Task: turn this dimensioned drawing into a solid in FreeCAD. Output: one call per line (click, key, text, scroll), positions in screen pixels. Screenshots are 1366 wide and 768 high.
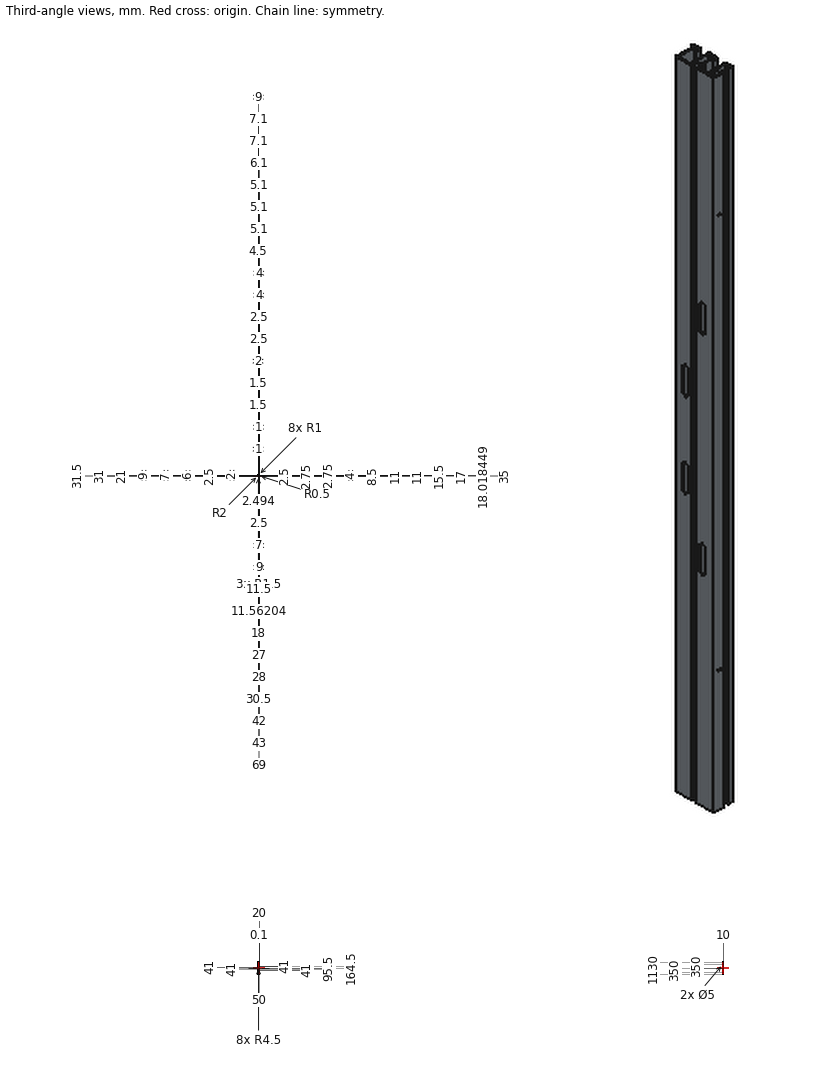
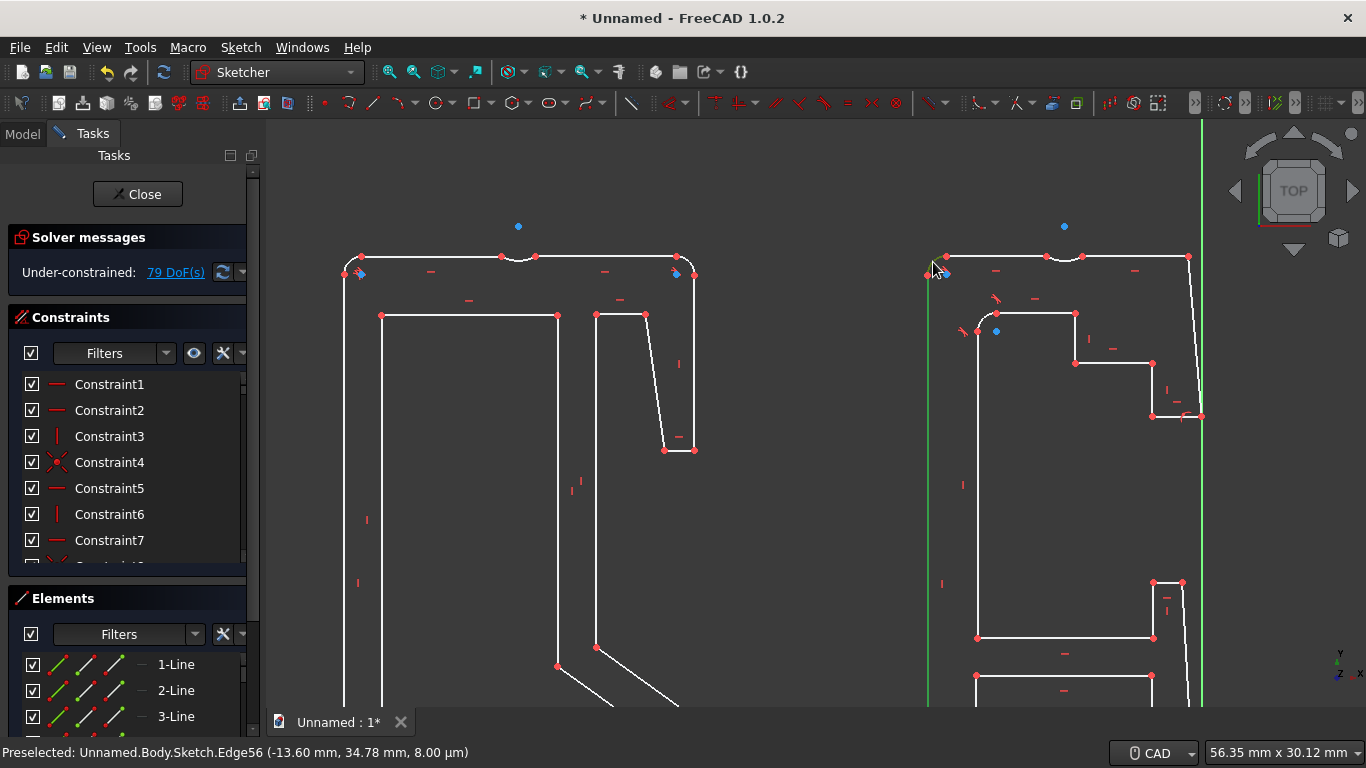
click(824, 104)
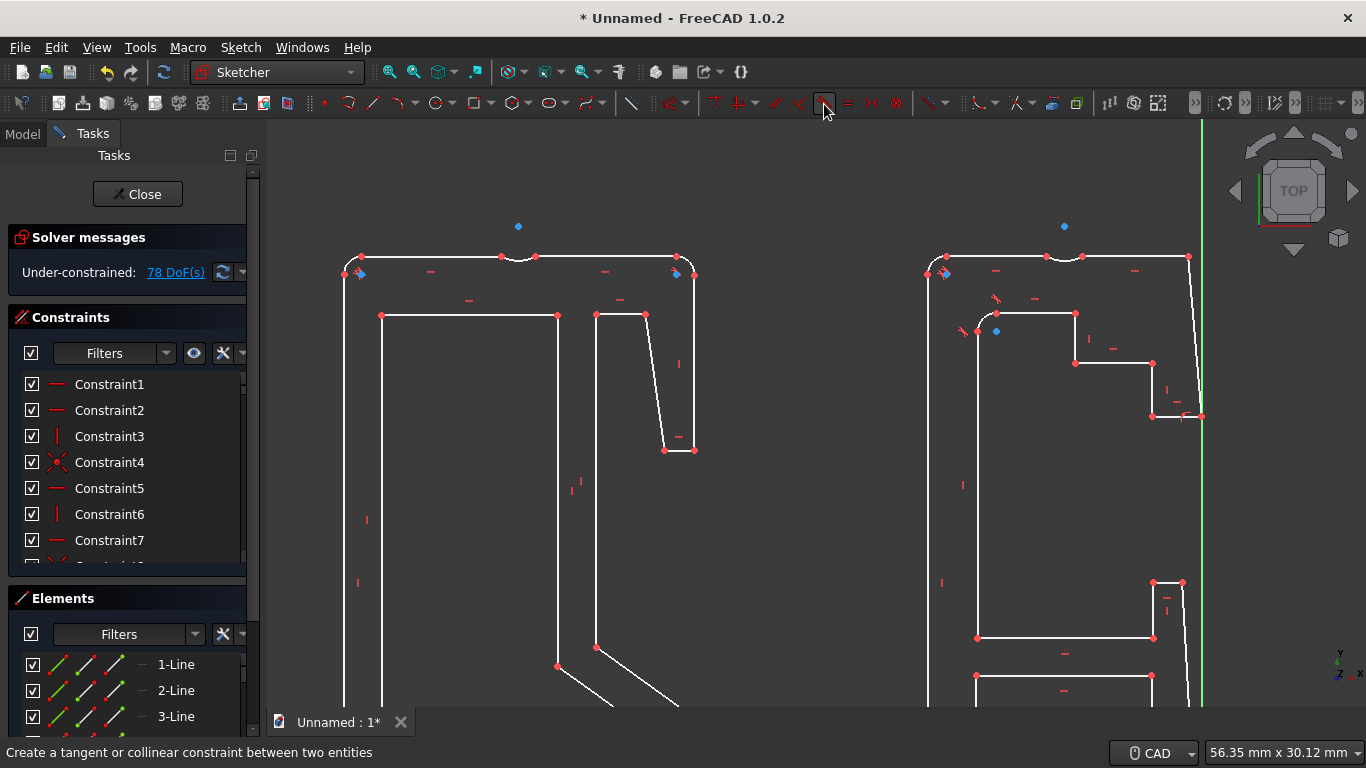
click(694, 398)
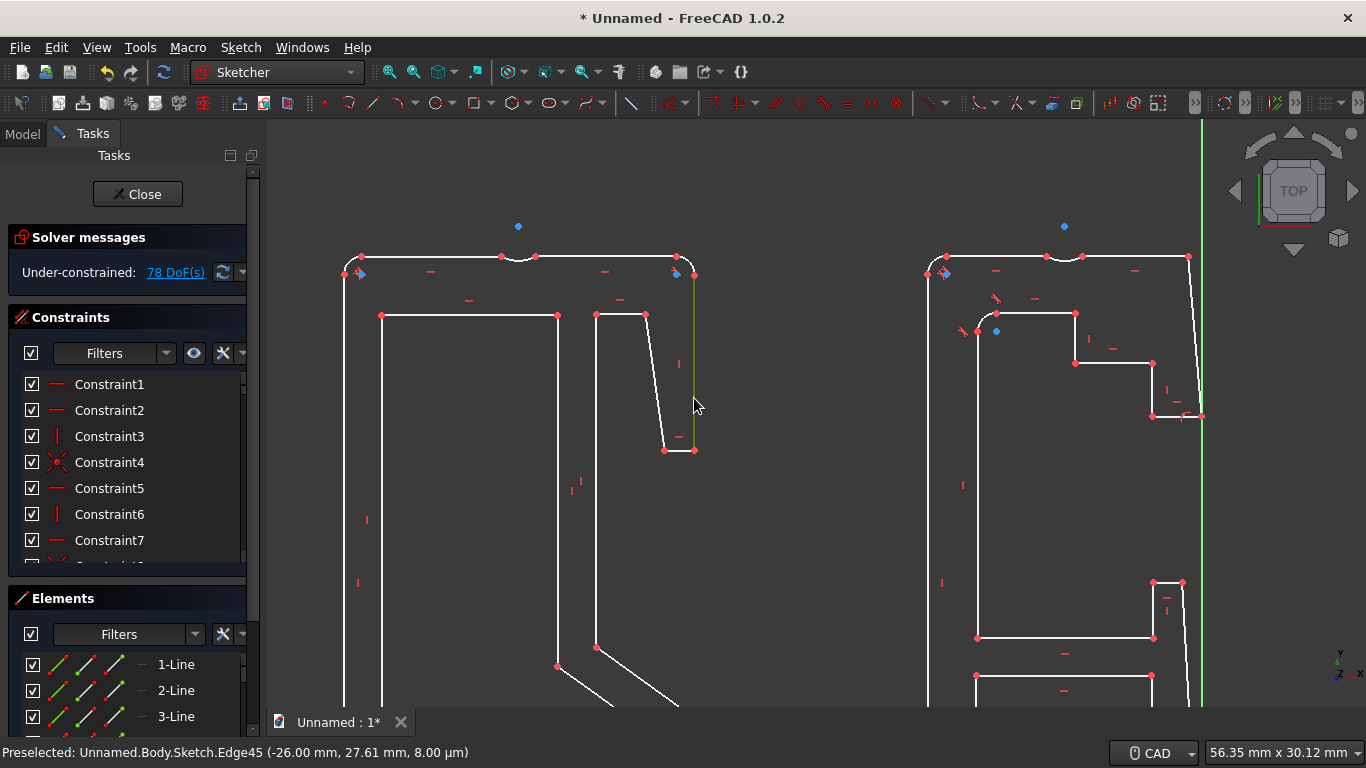
click(690, 262)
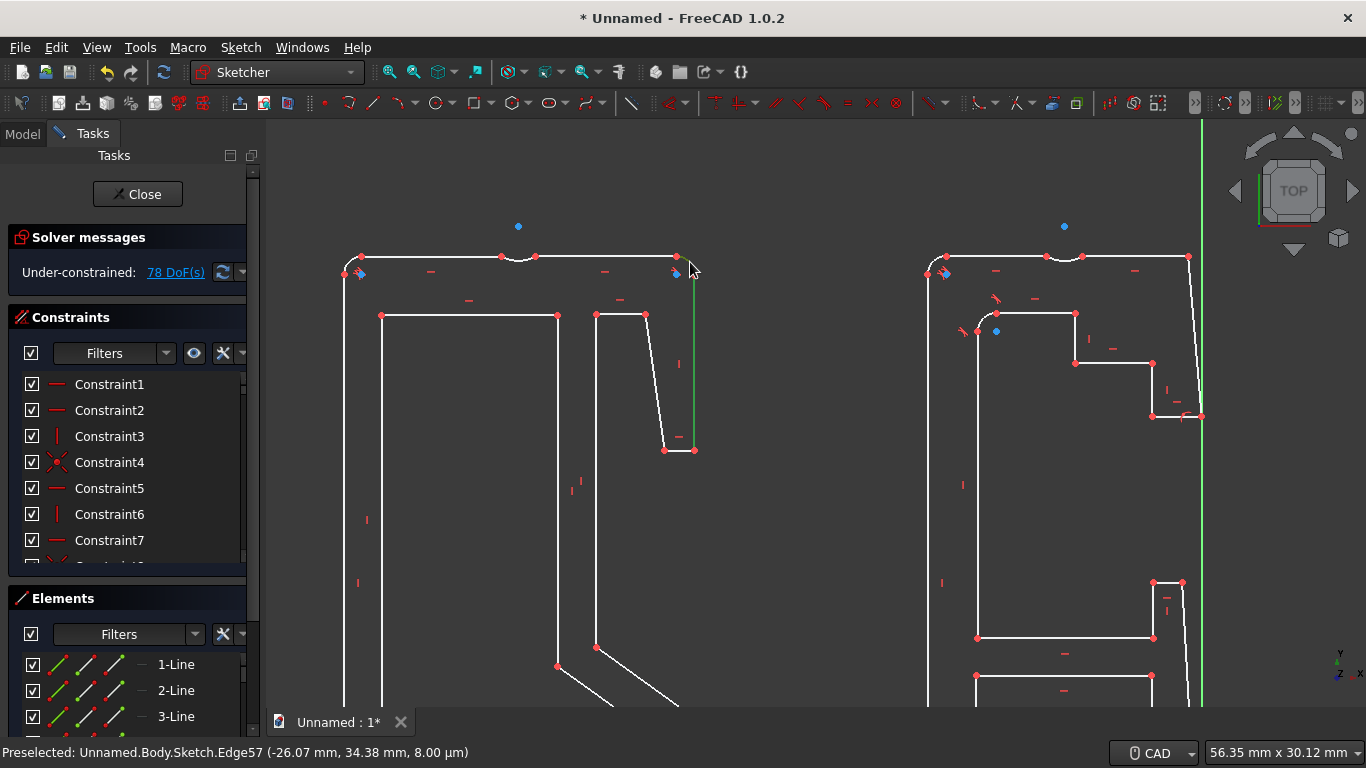
key(t)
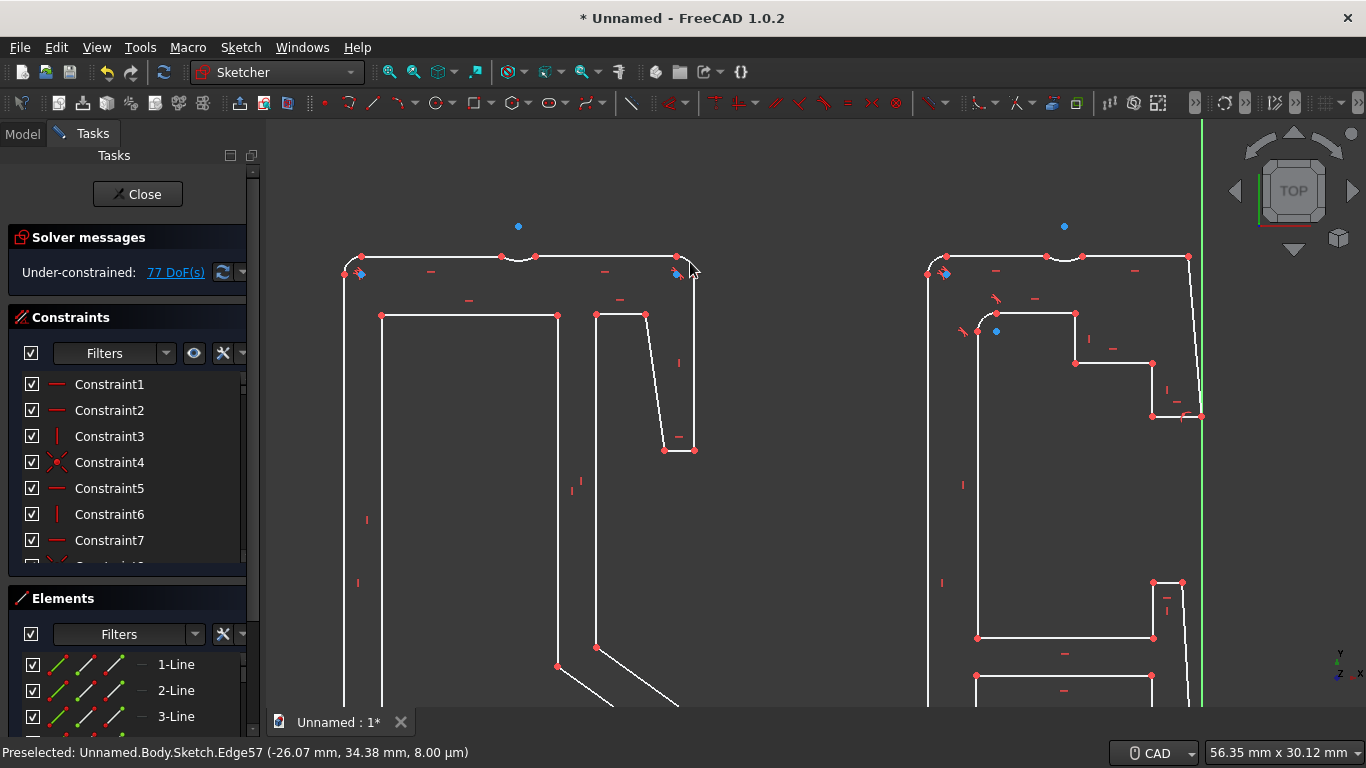
scroll(934, 263, down, 4)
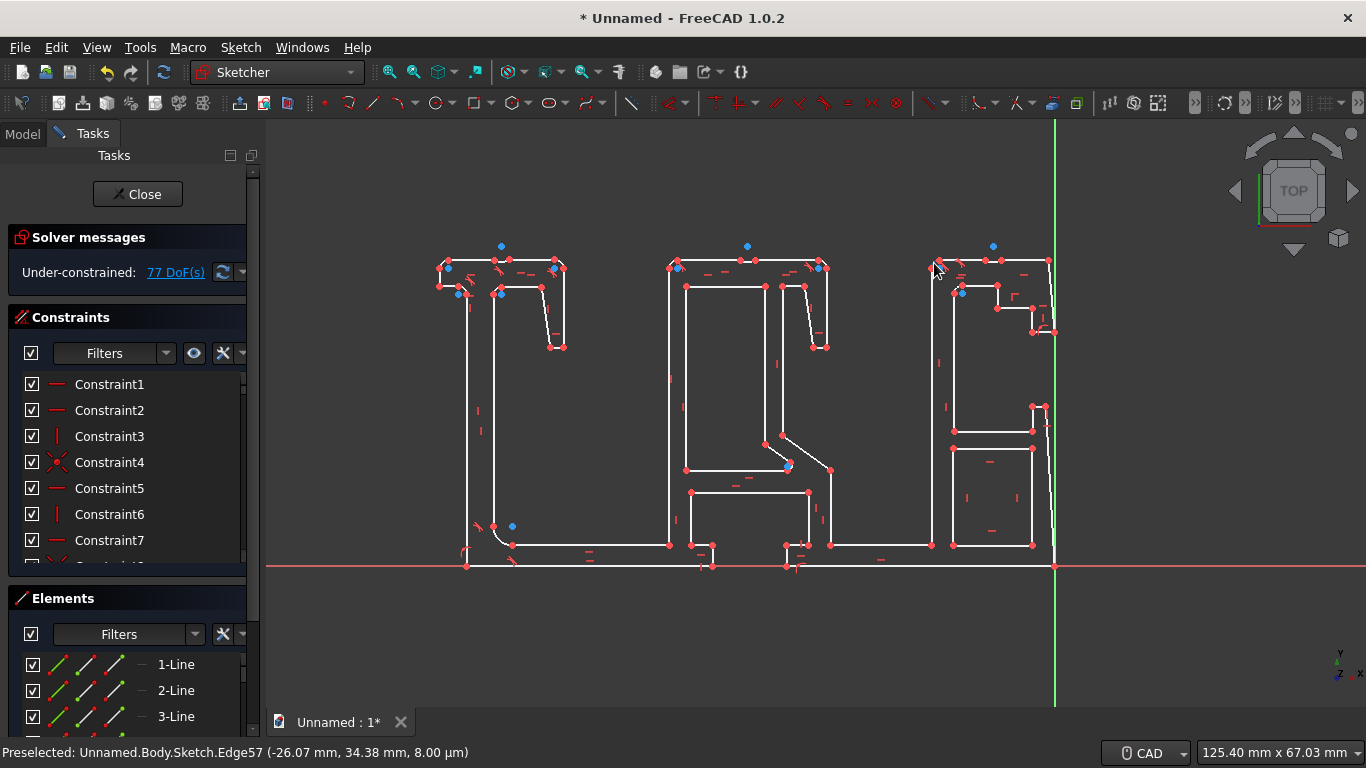
click(757, 471)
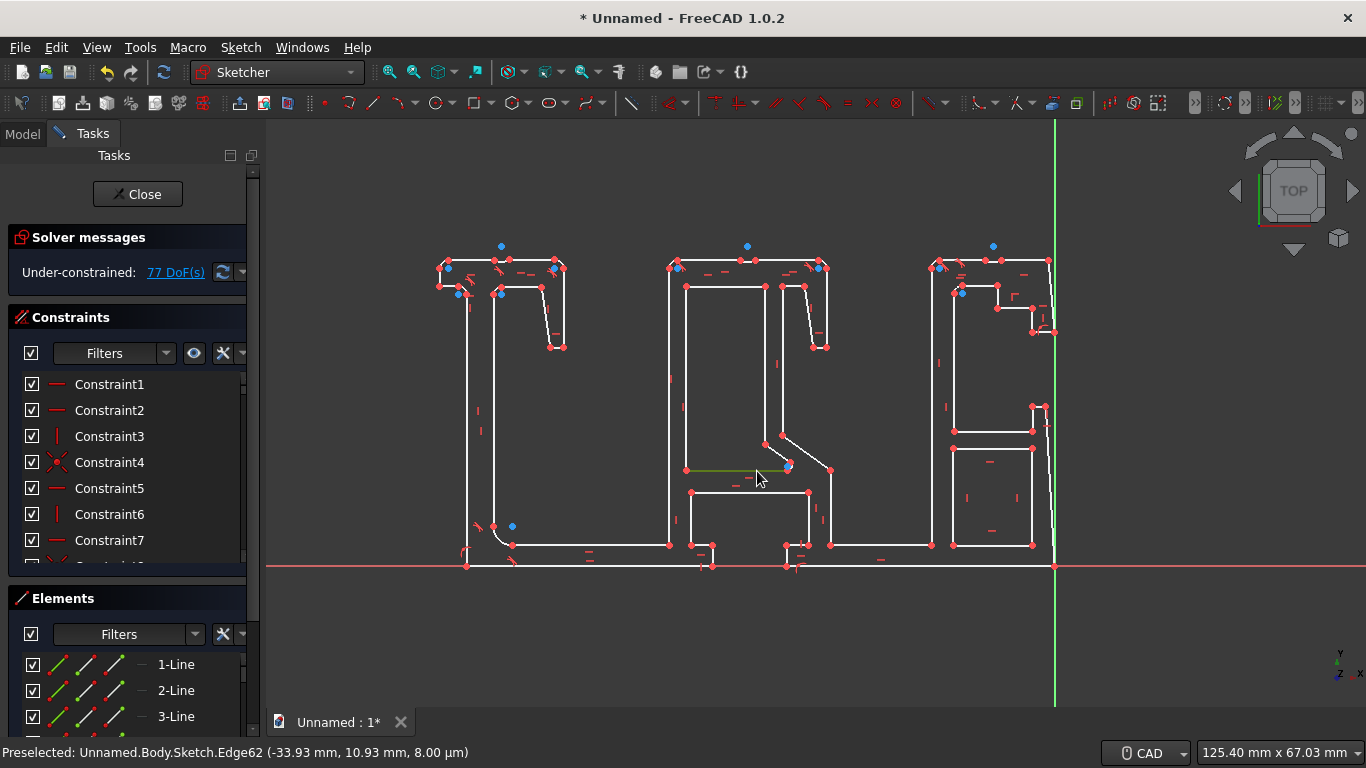
scroll(792, 467, up, 6)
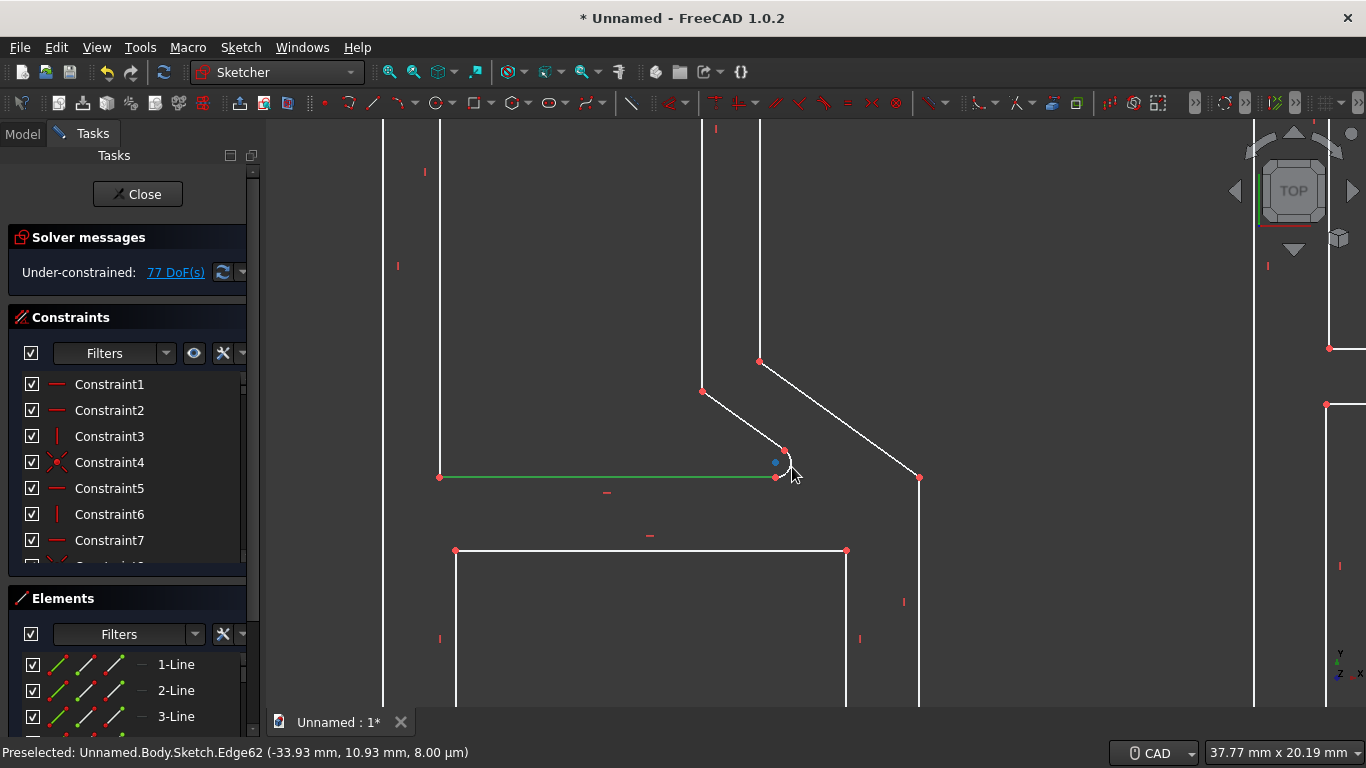
click(790, 467)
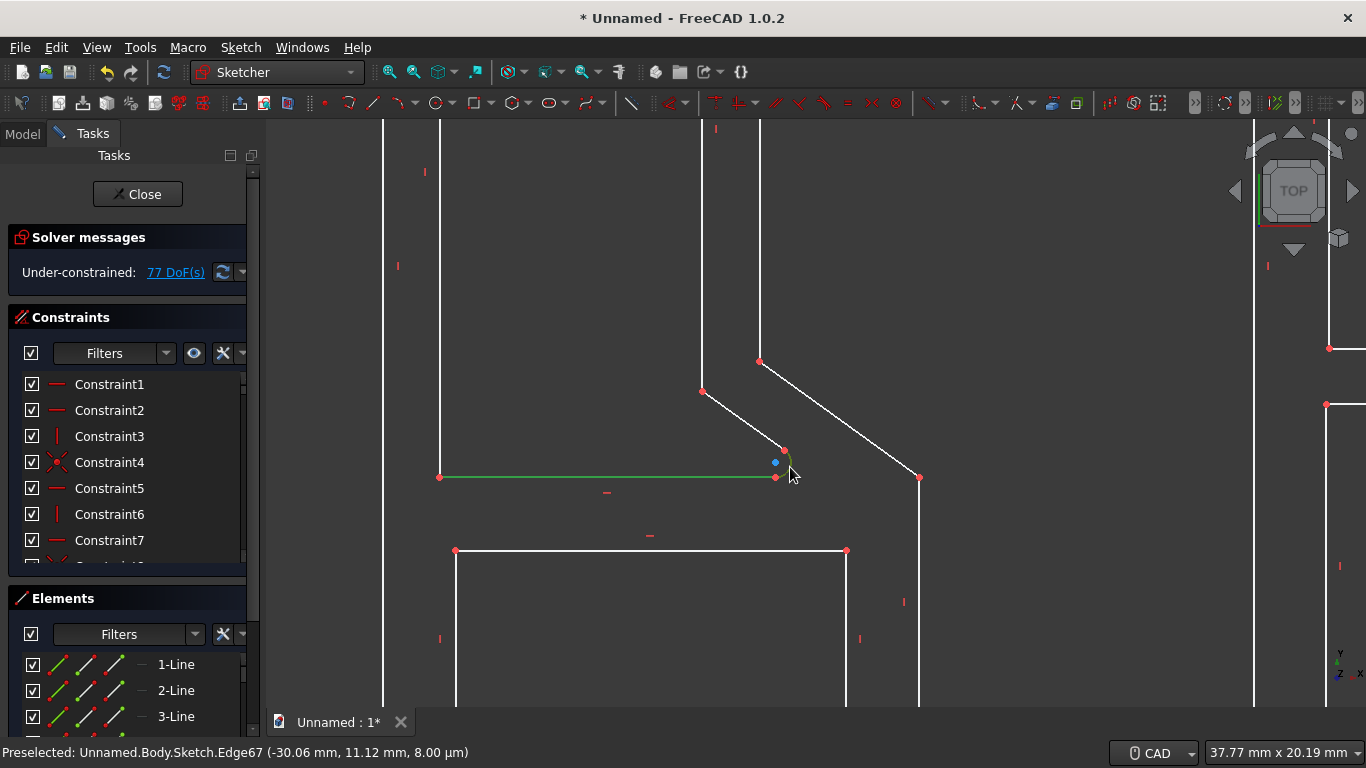
key(t)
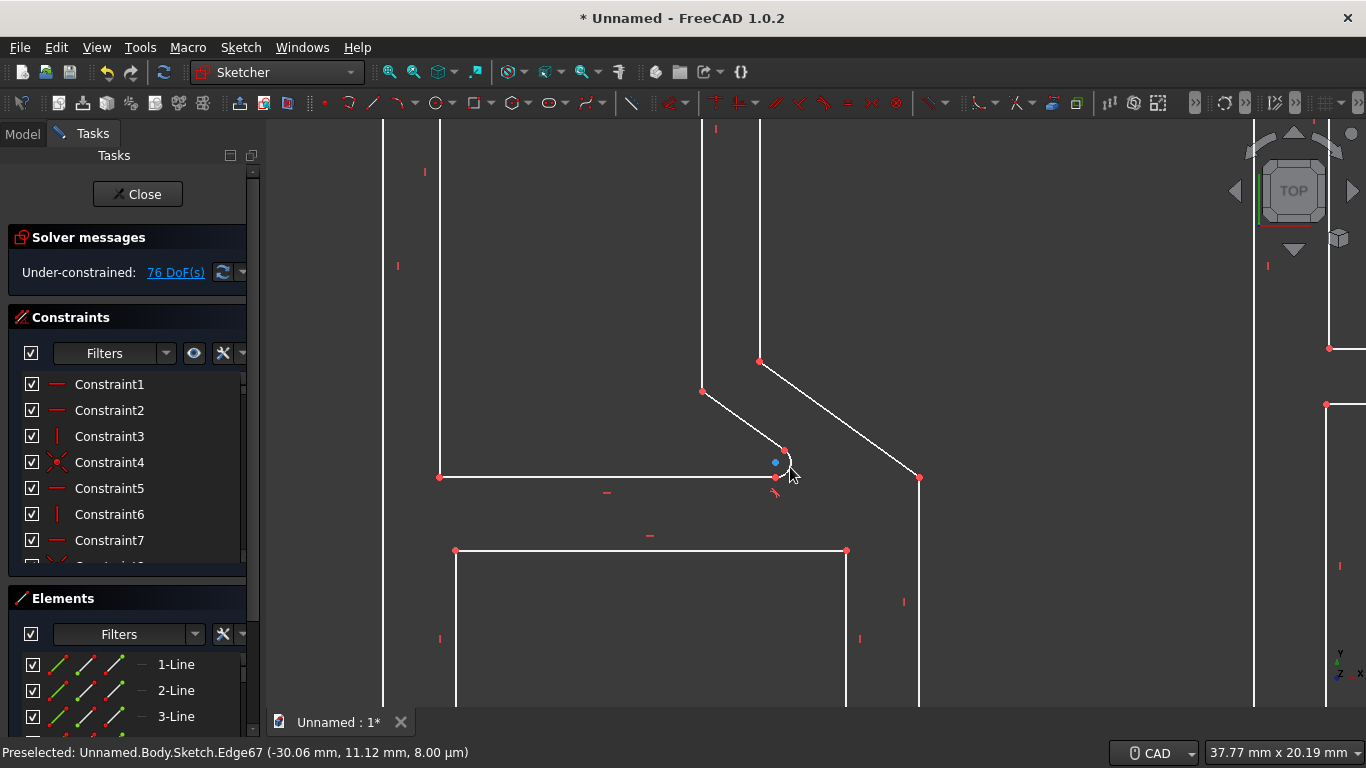
click(727, 409)